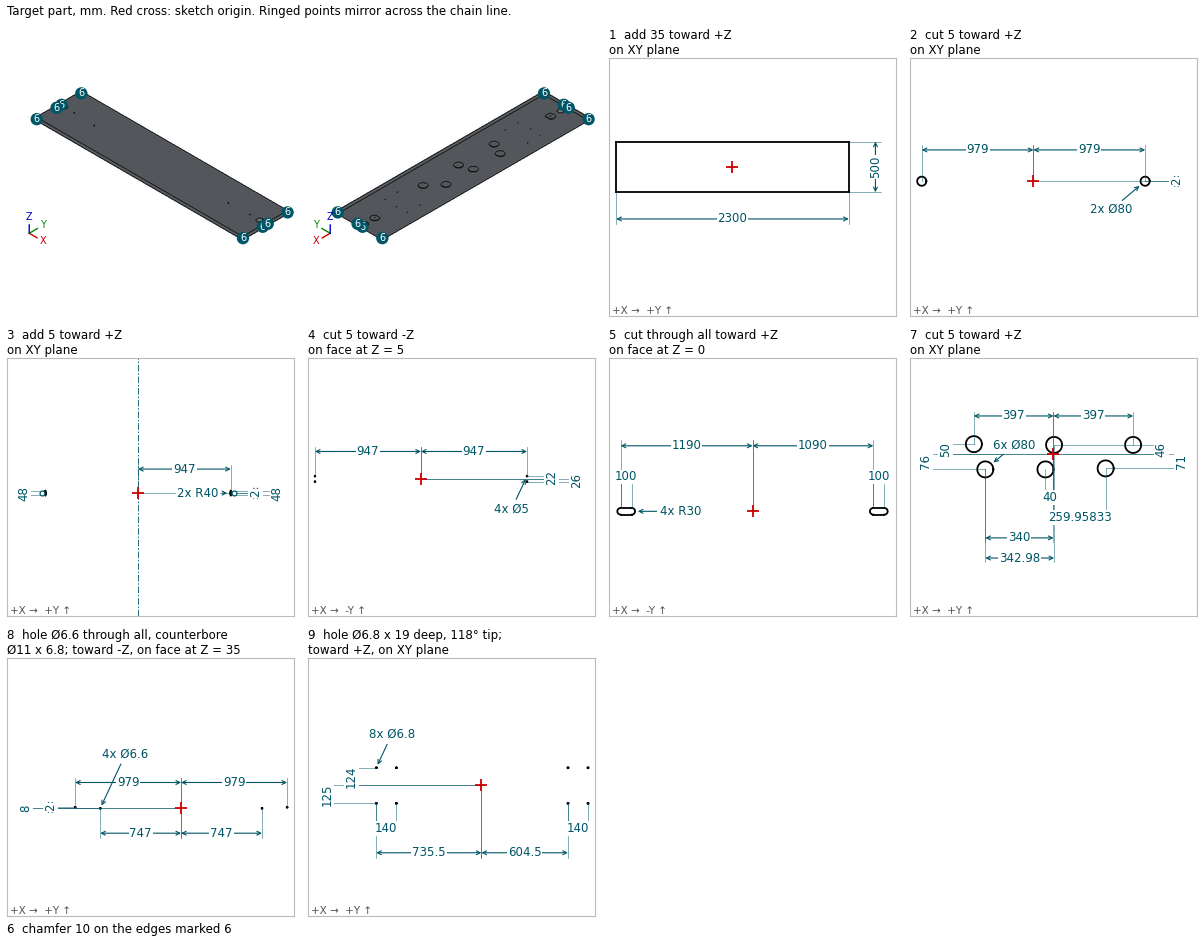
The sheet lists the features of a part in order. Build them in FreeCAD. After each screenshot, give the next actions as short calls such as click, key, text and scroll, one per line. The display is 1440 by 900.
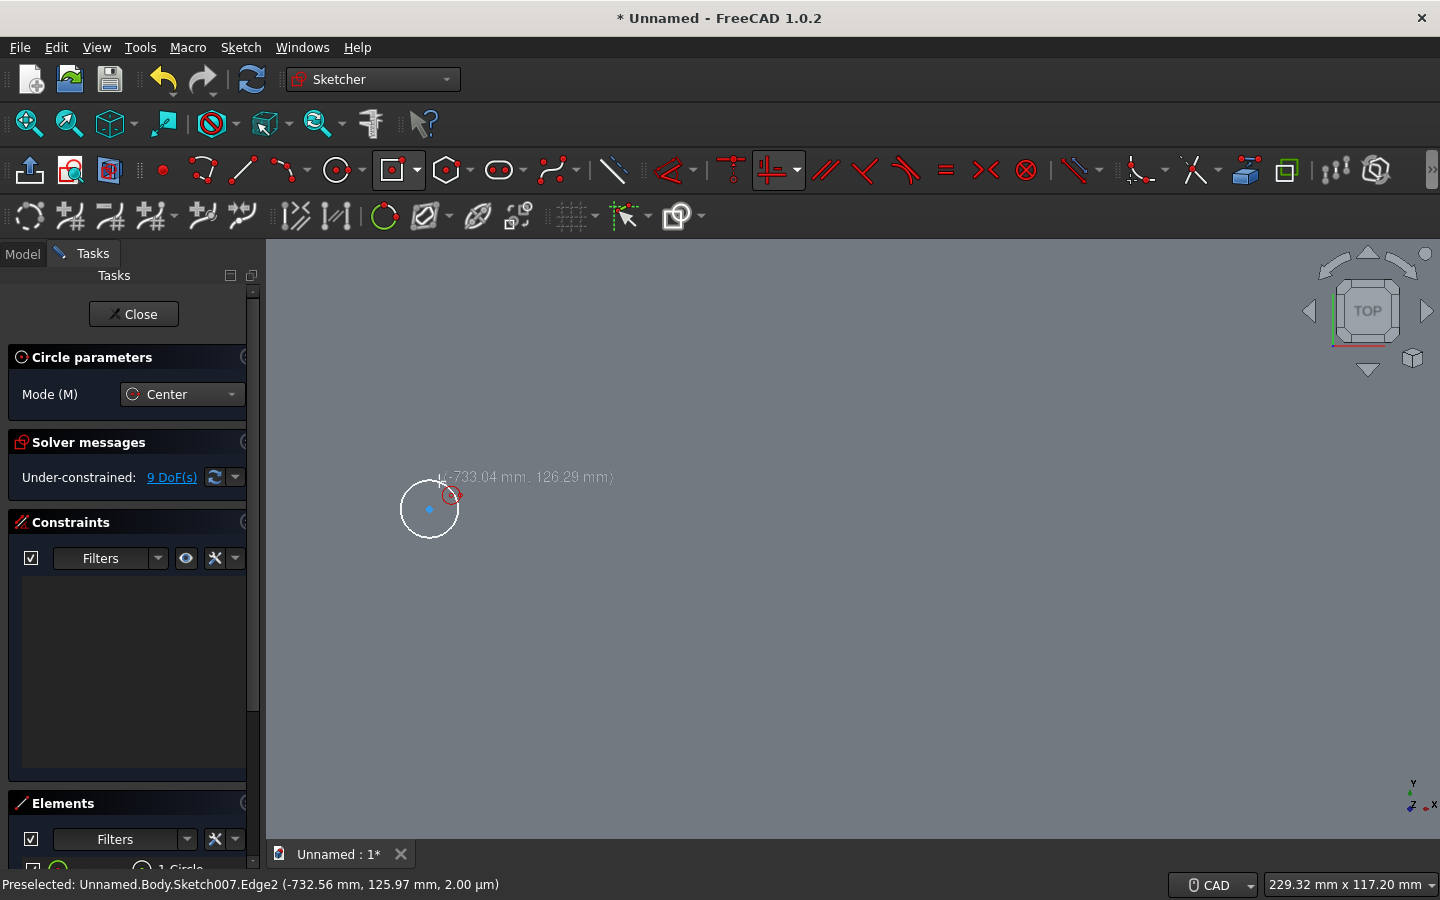
scroll(1143, 494, up, 2)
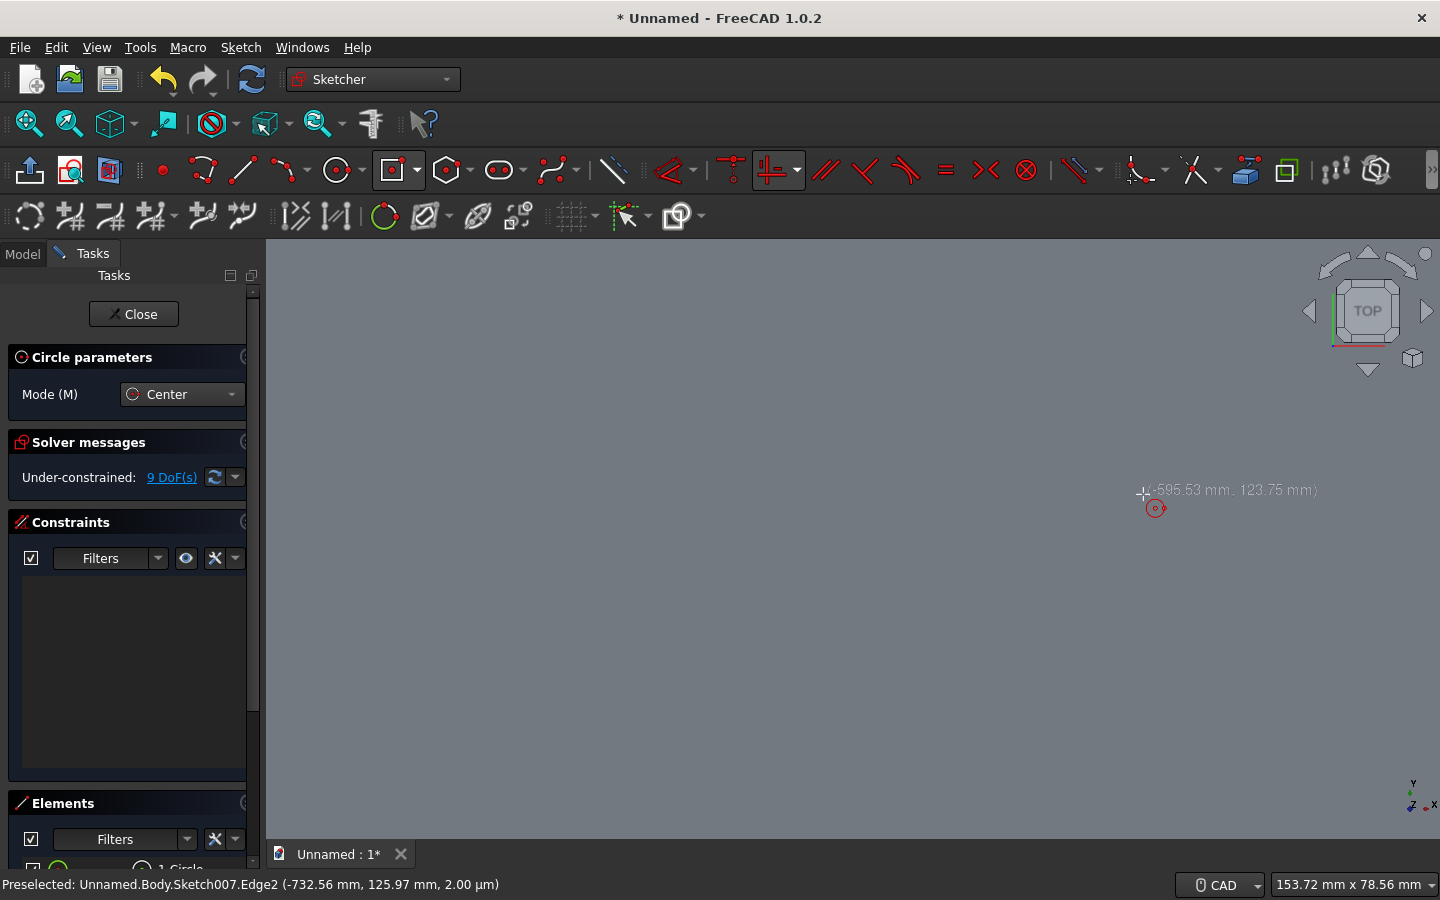
scroll(465, 480, down, 14)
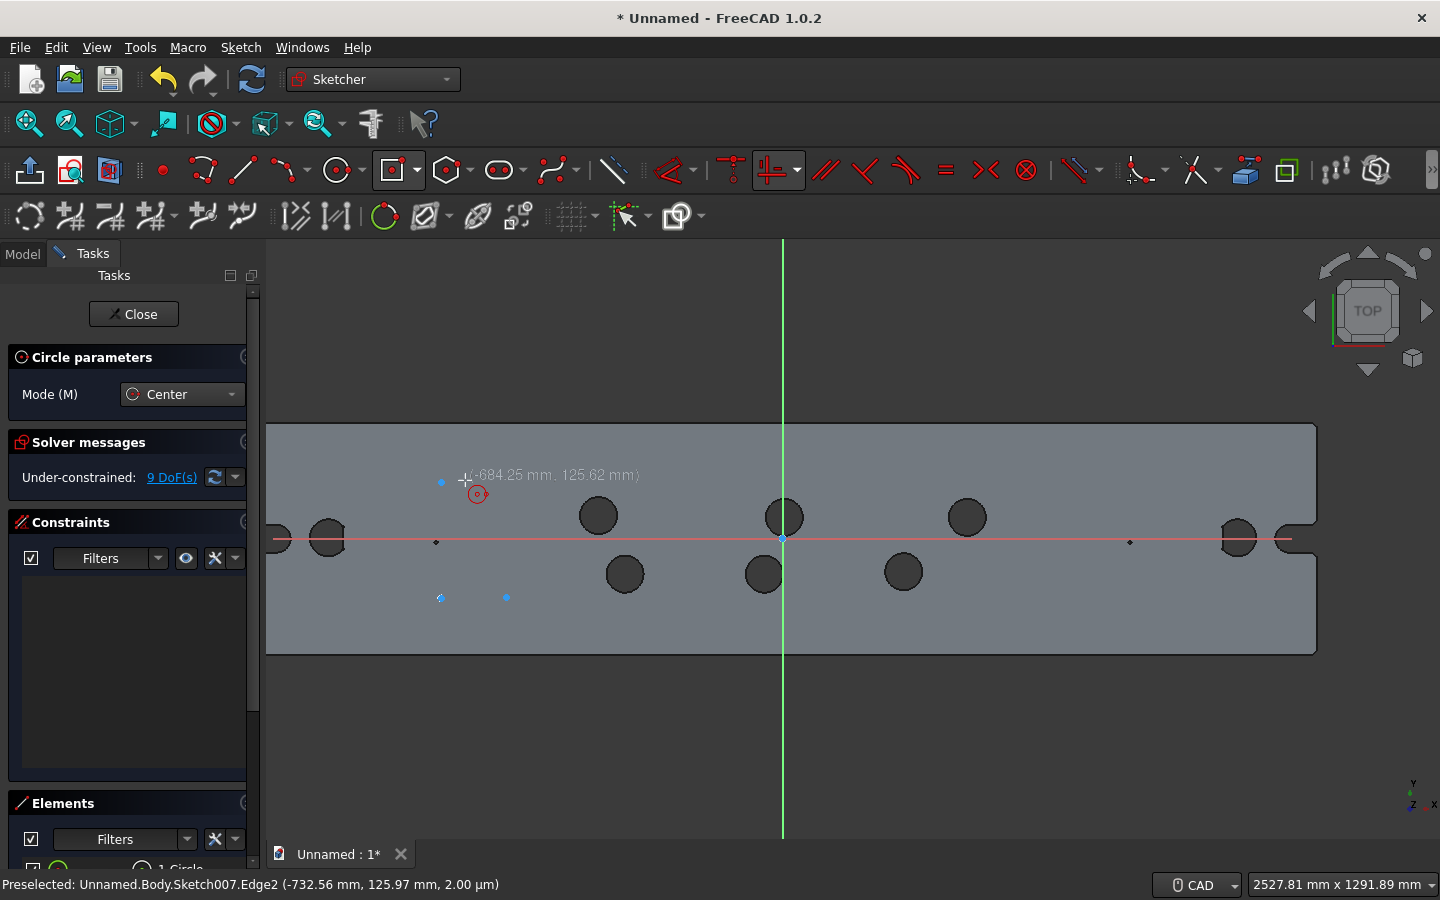
click(506, 481)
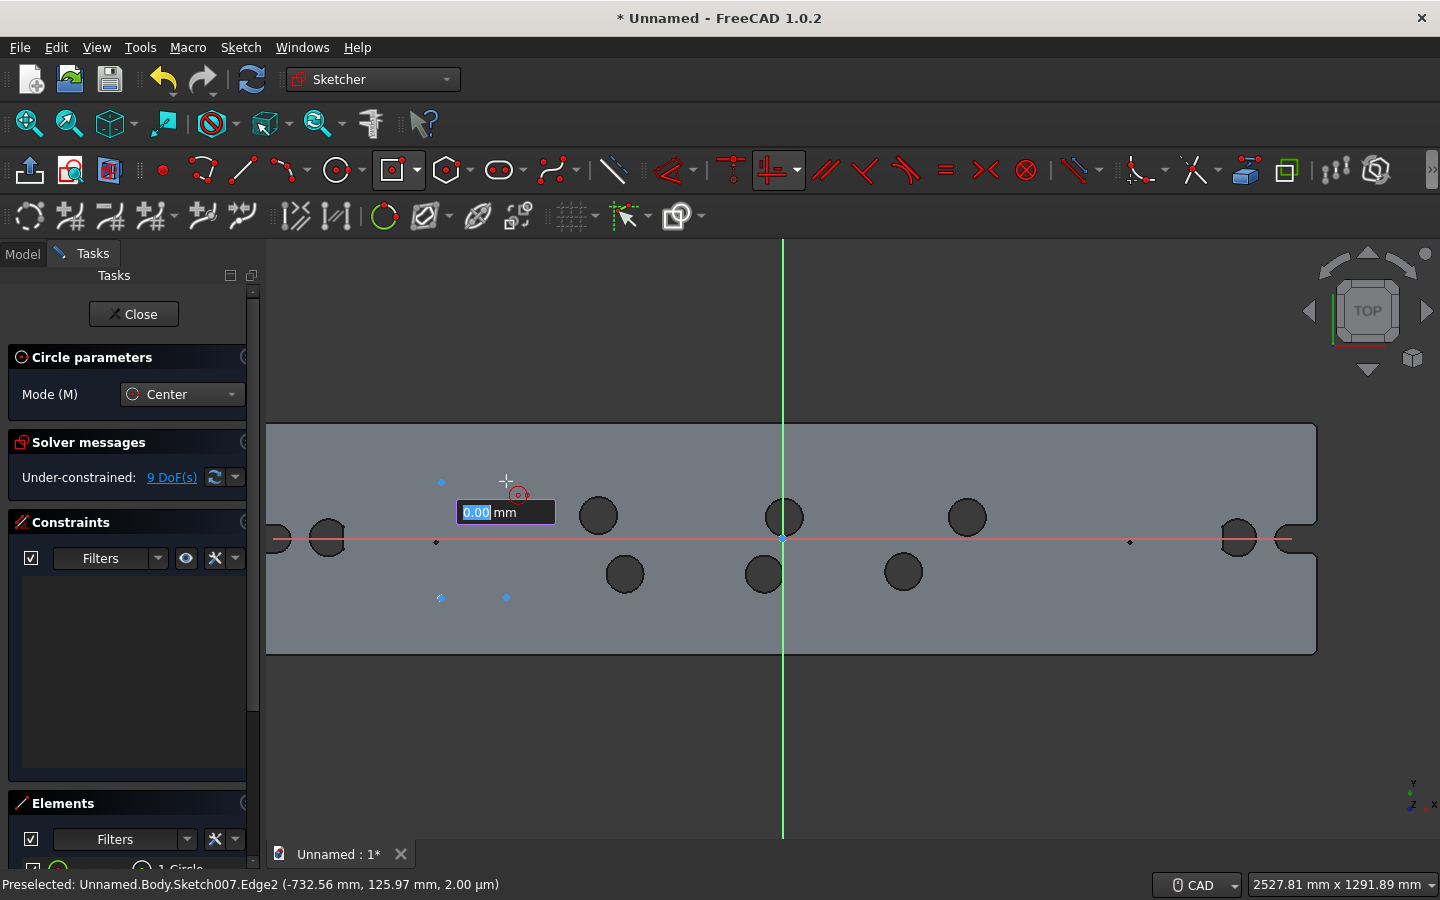
scroll(507, 480, up, 12)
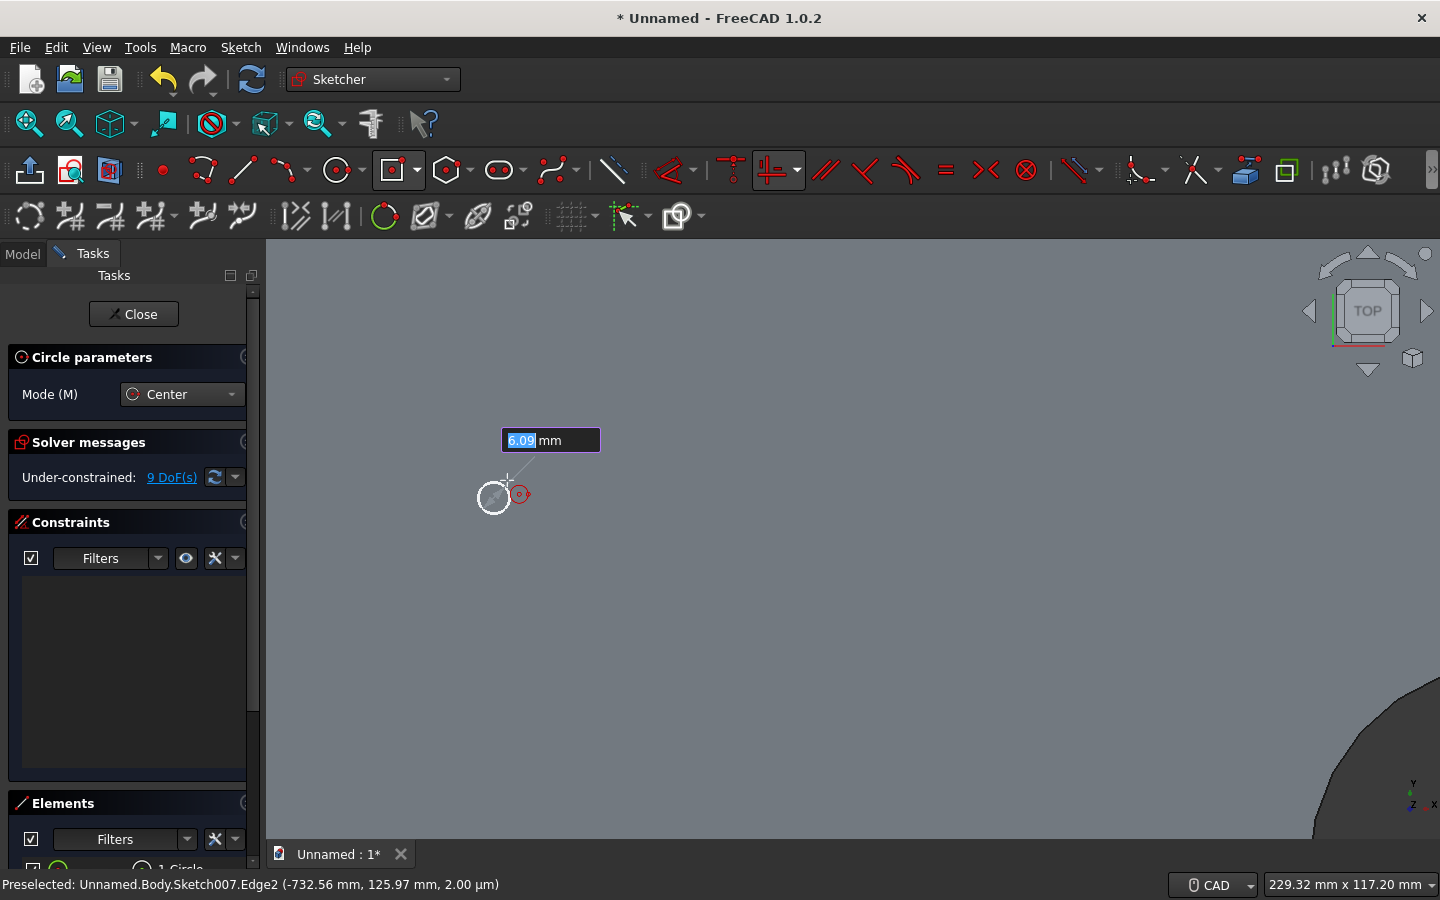
click(510, 477)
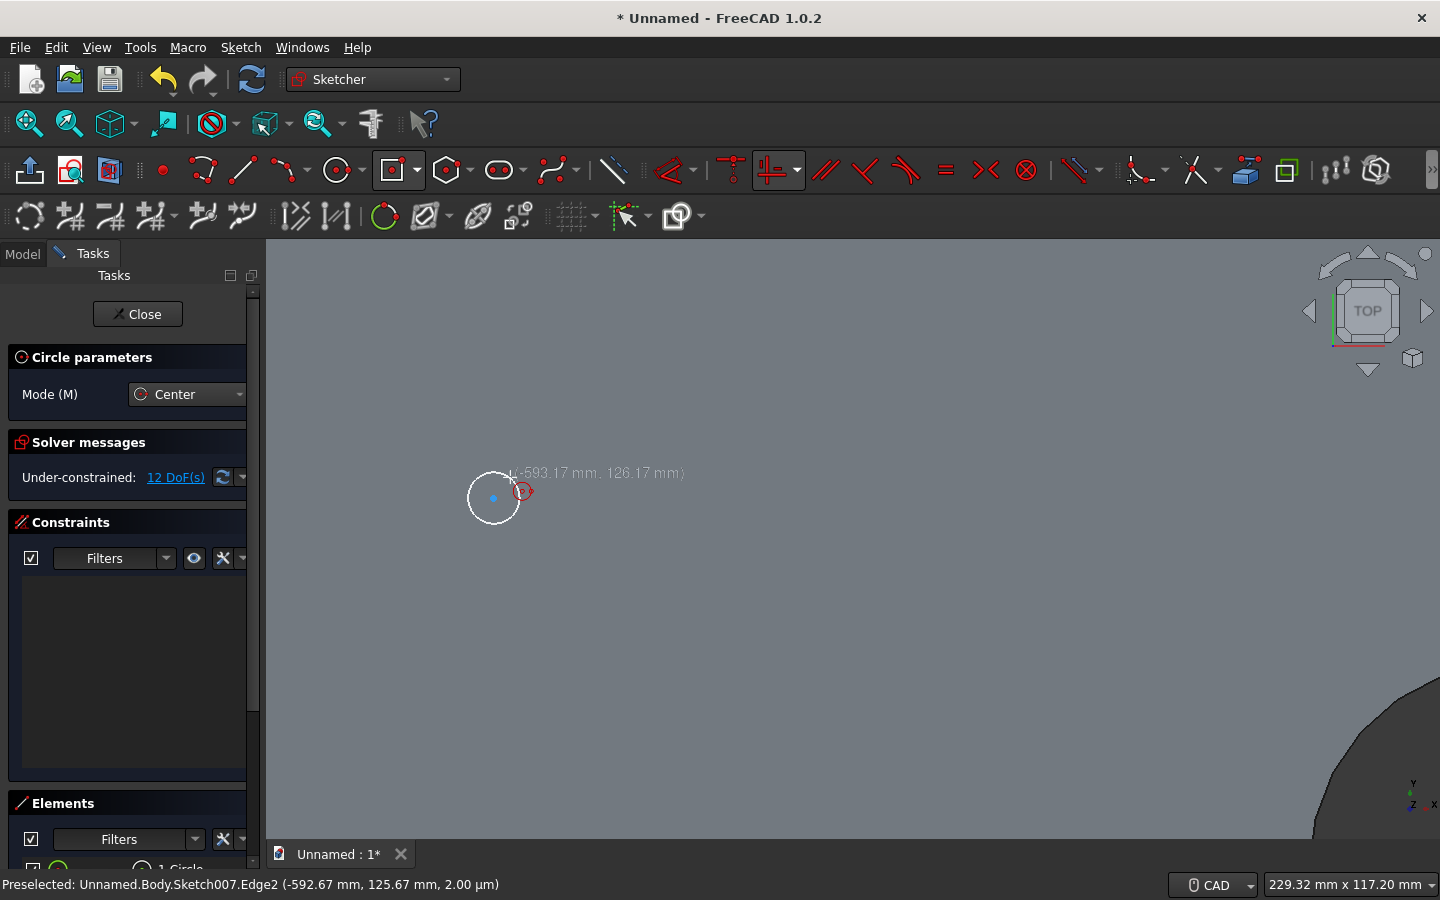
scroll(507, 480, down, 12)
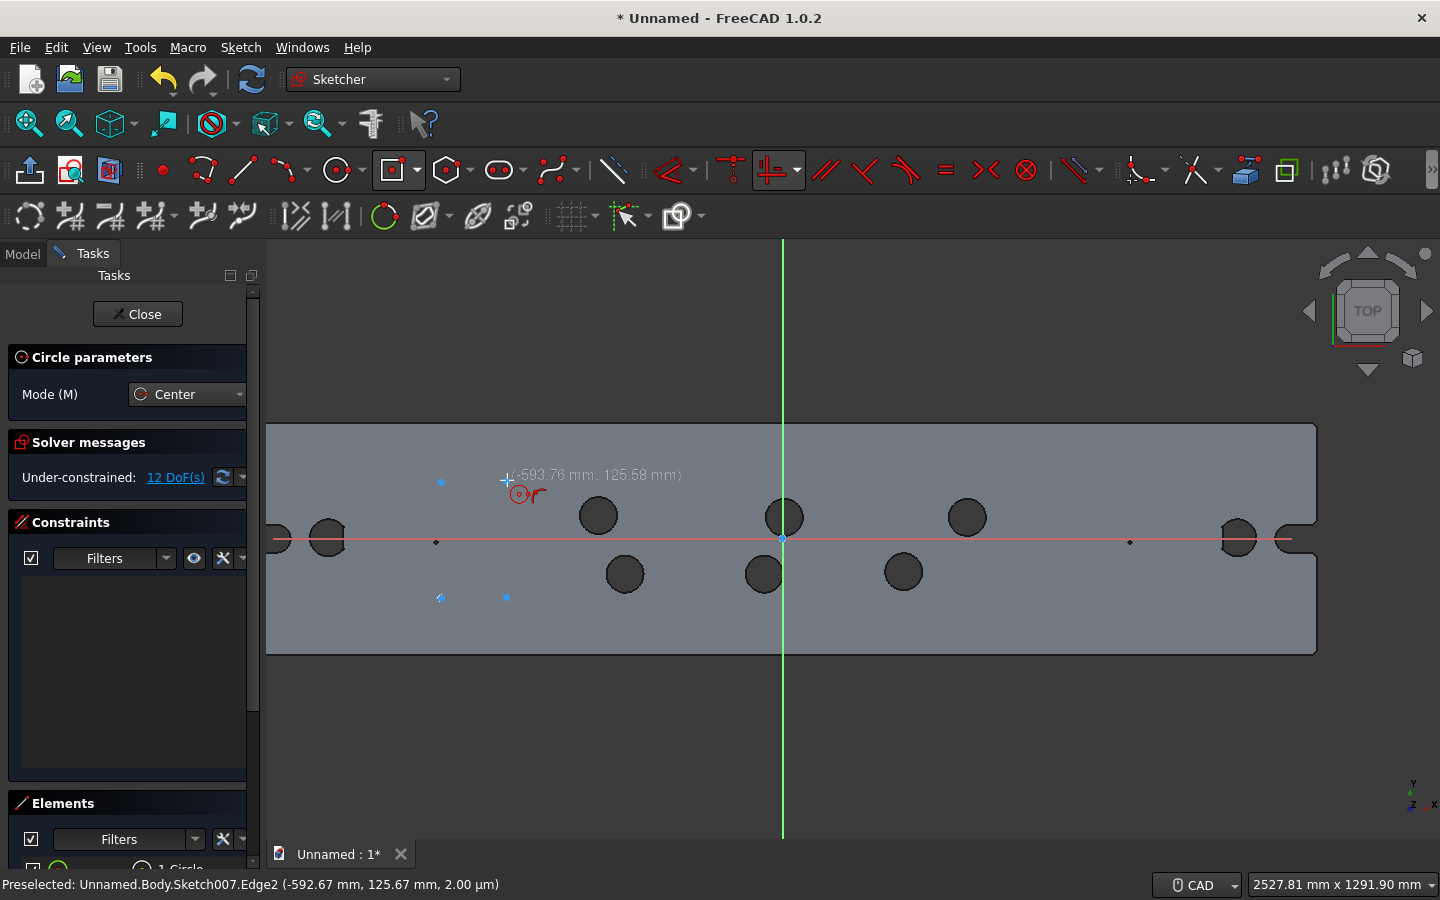
scroll(1064, 597, up, 14)